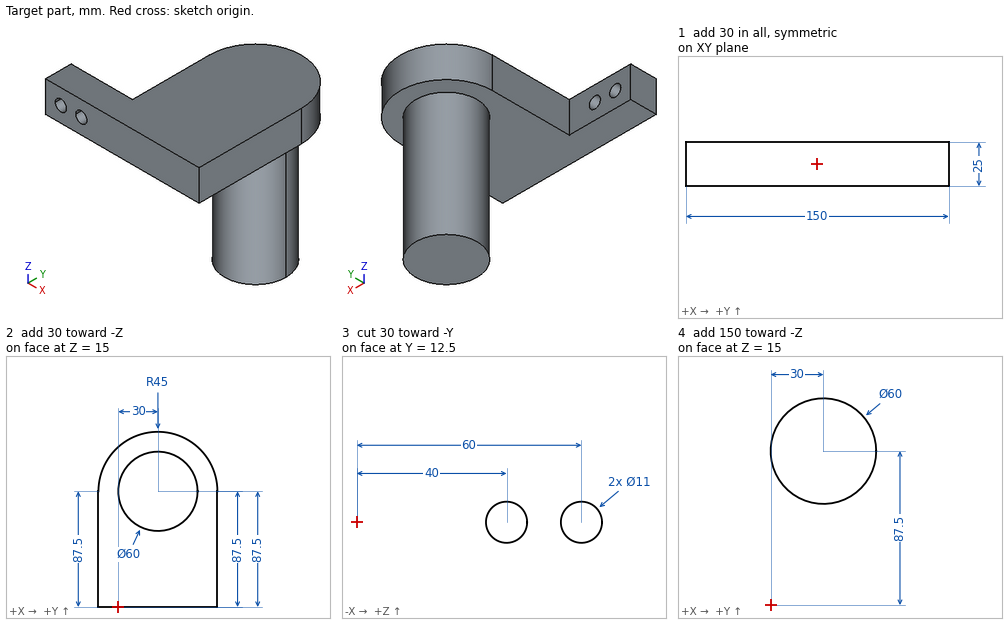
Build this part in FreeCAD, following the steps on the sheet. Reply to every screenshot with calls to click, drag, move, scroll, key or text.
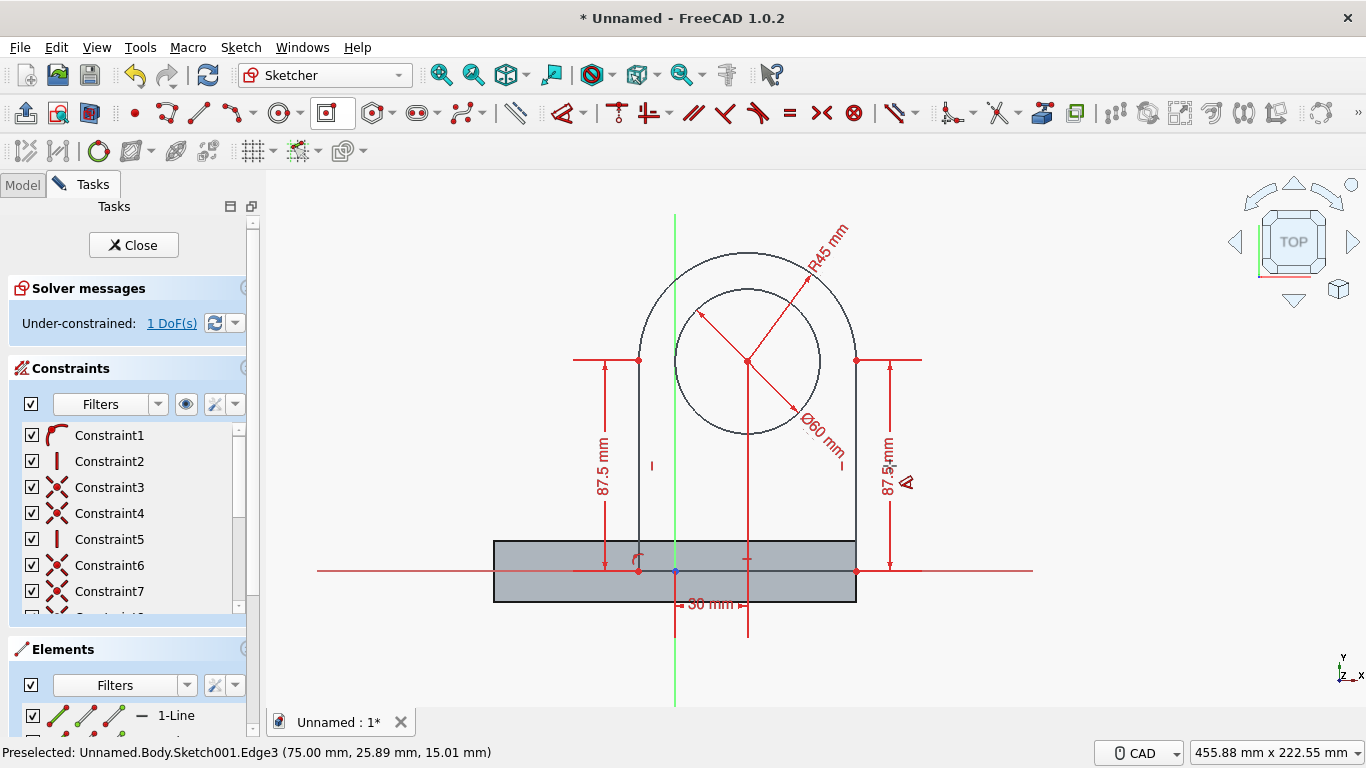
click(748, 361)
click(782, 466)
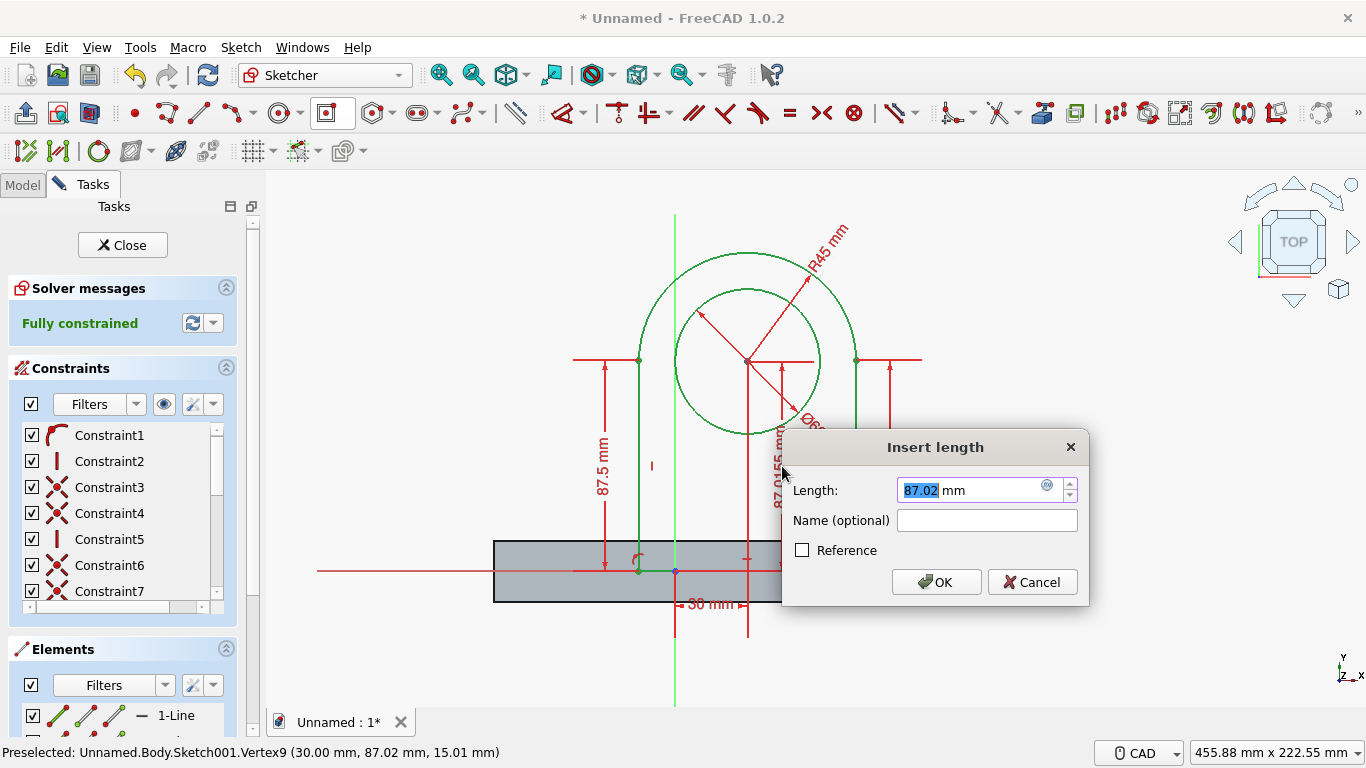
text(87.5)
key(Return)
key(Escape)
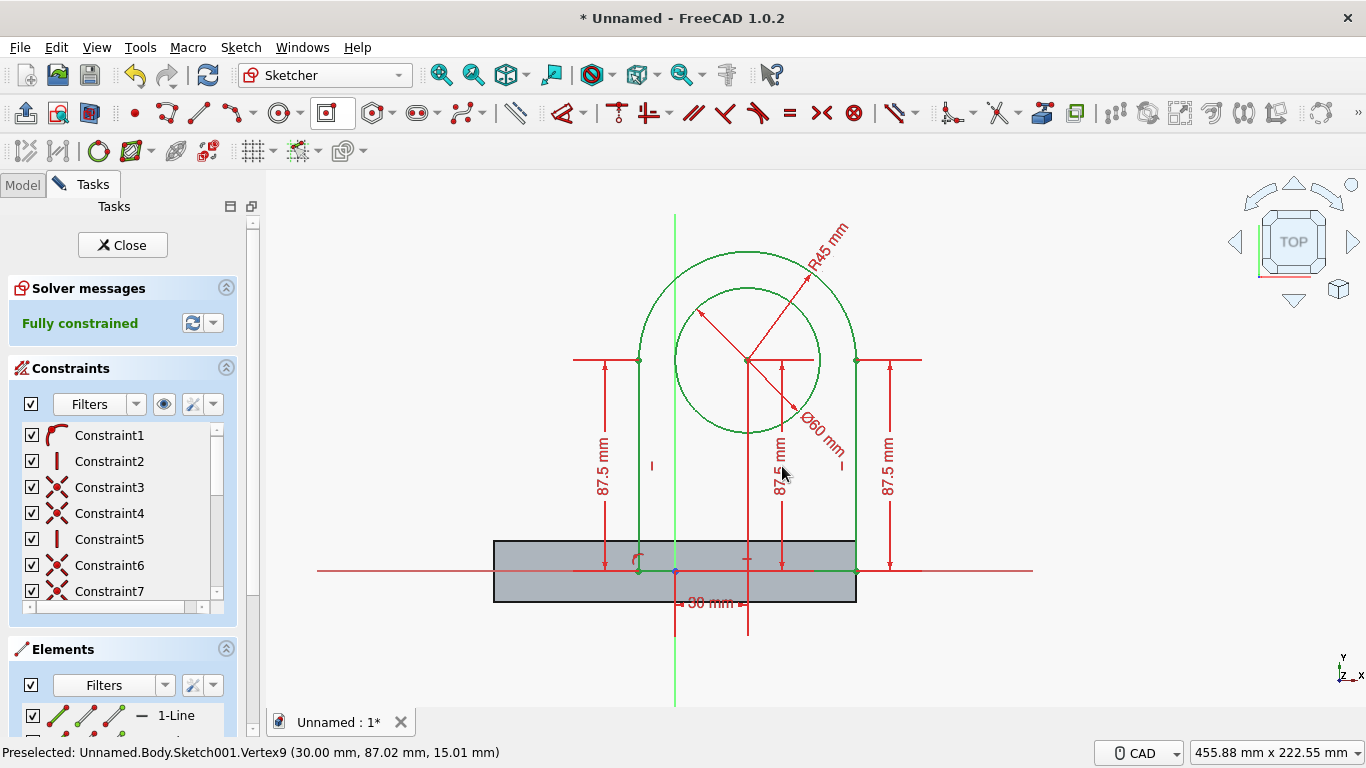
click(123, 245)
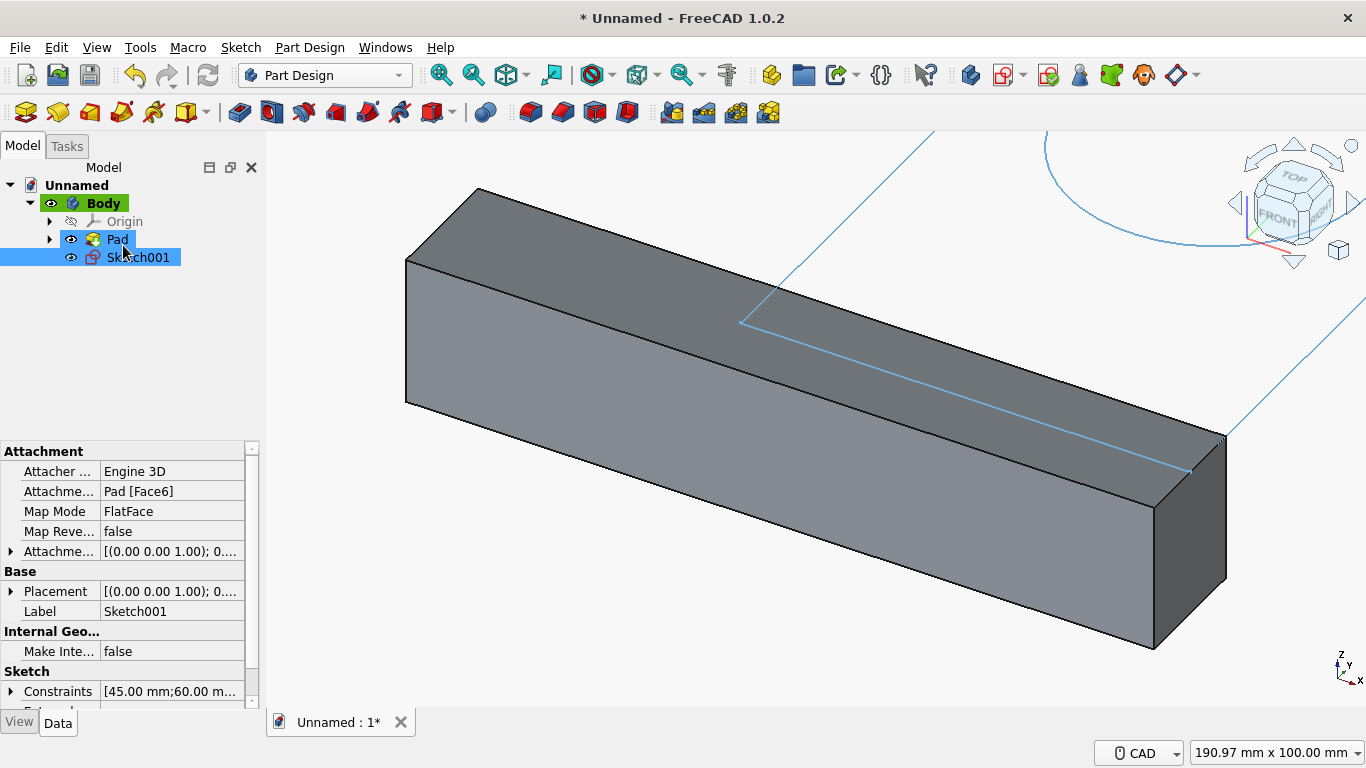
click(26, 112)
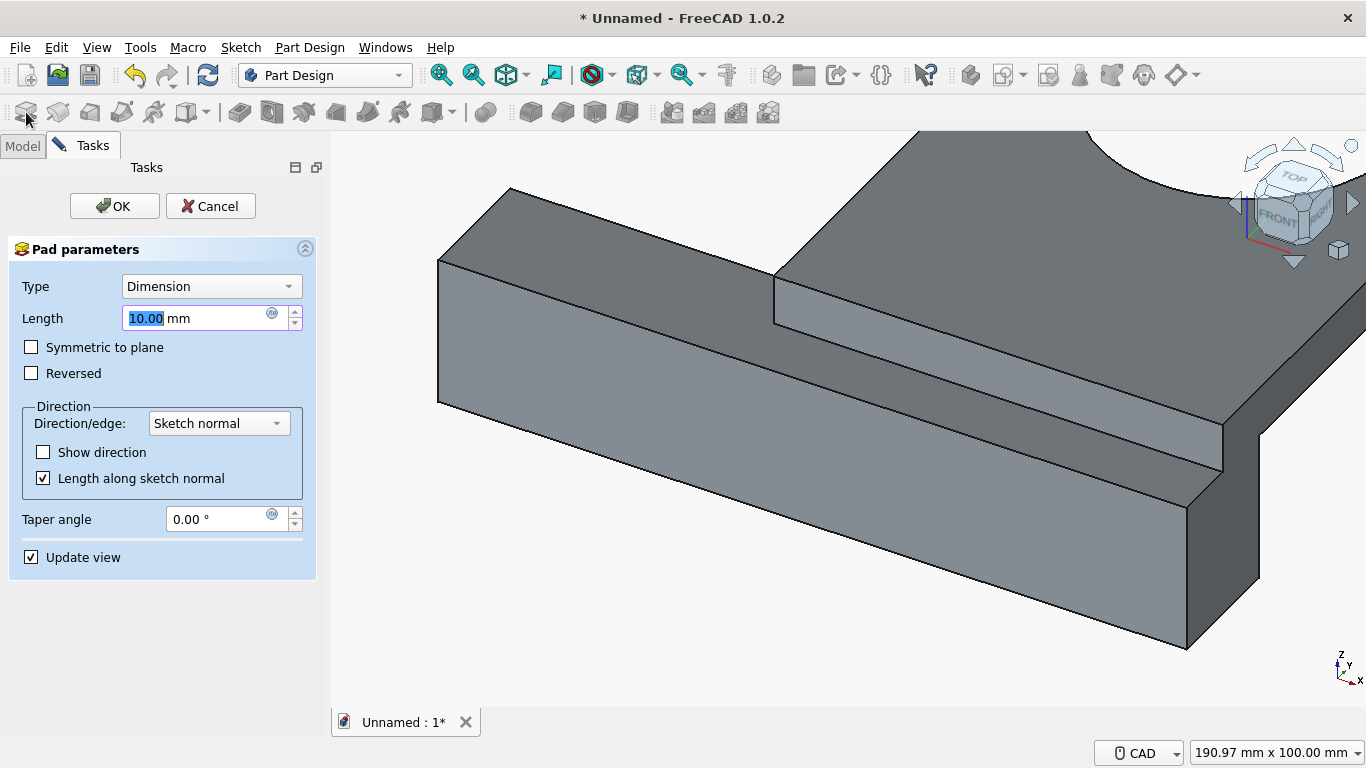
text(30)
key(Tab)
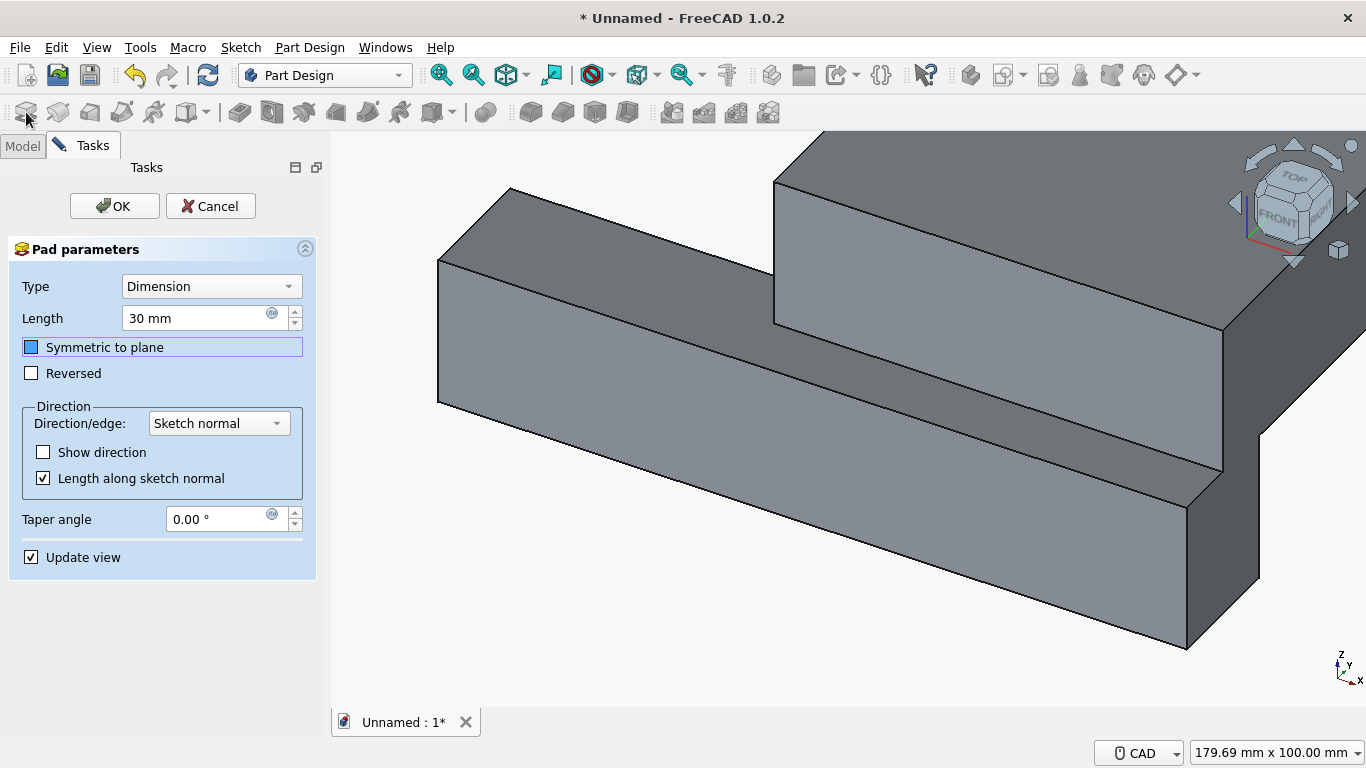
click(30, 373)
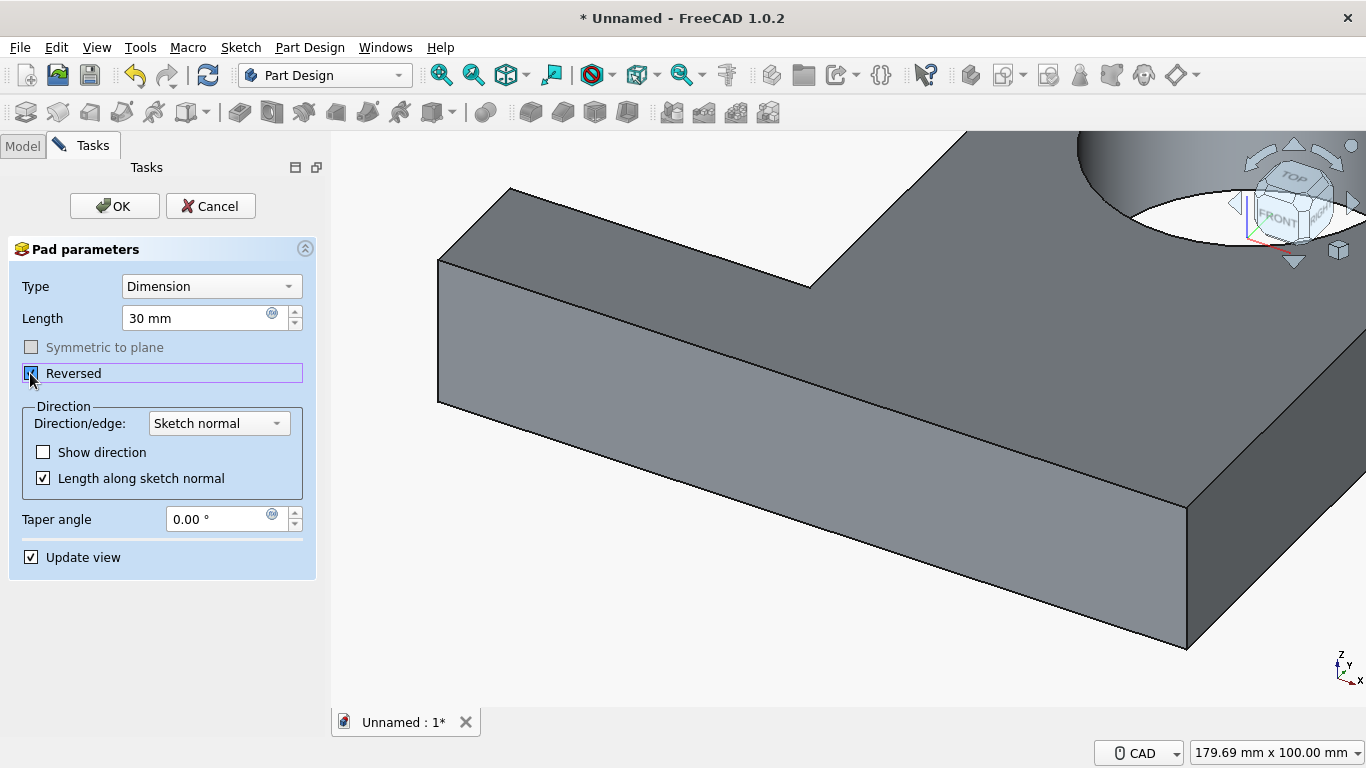
click(115, 206)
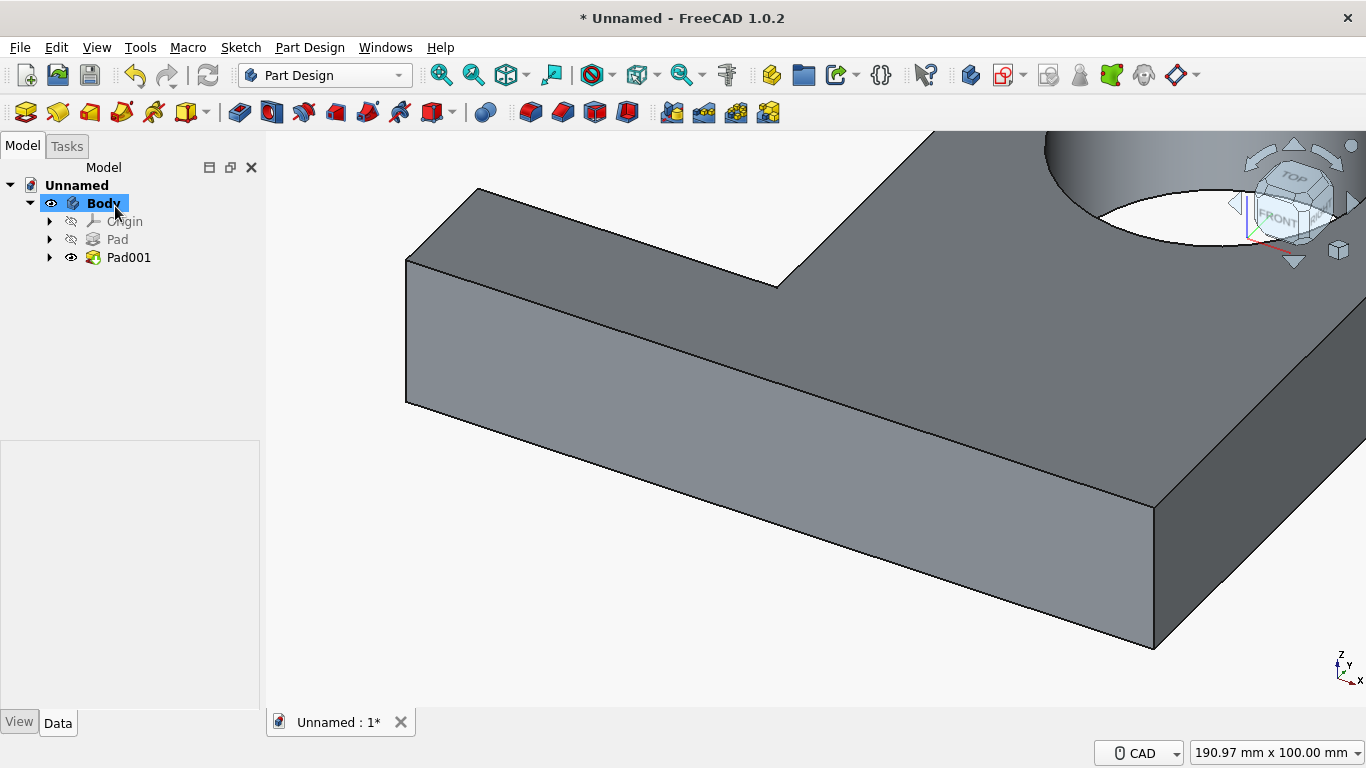
click(442, 76)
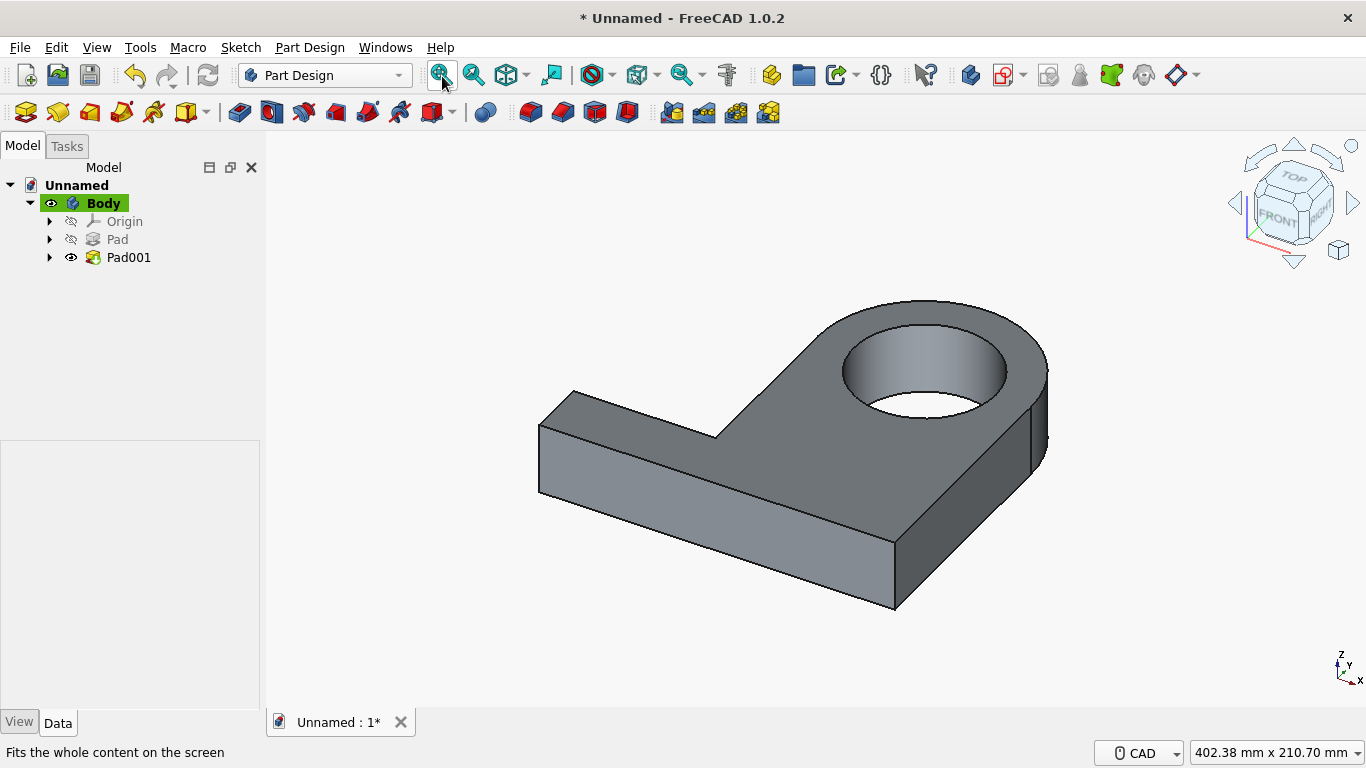
key(4)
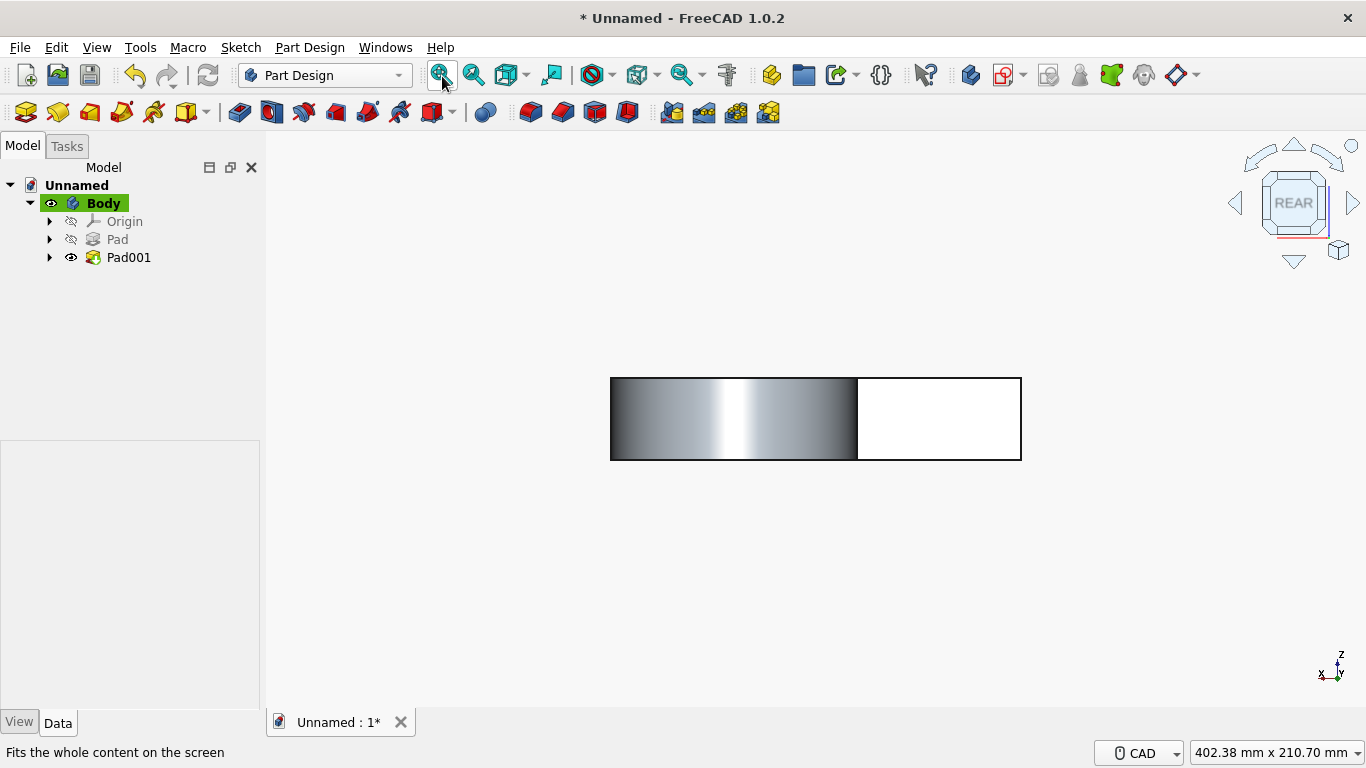
key(v)
key(f)